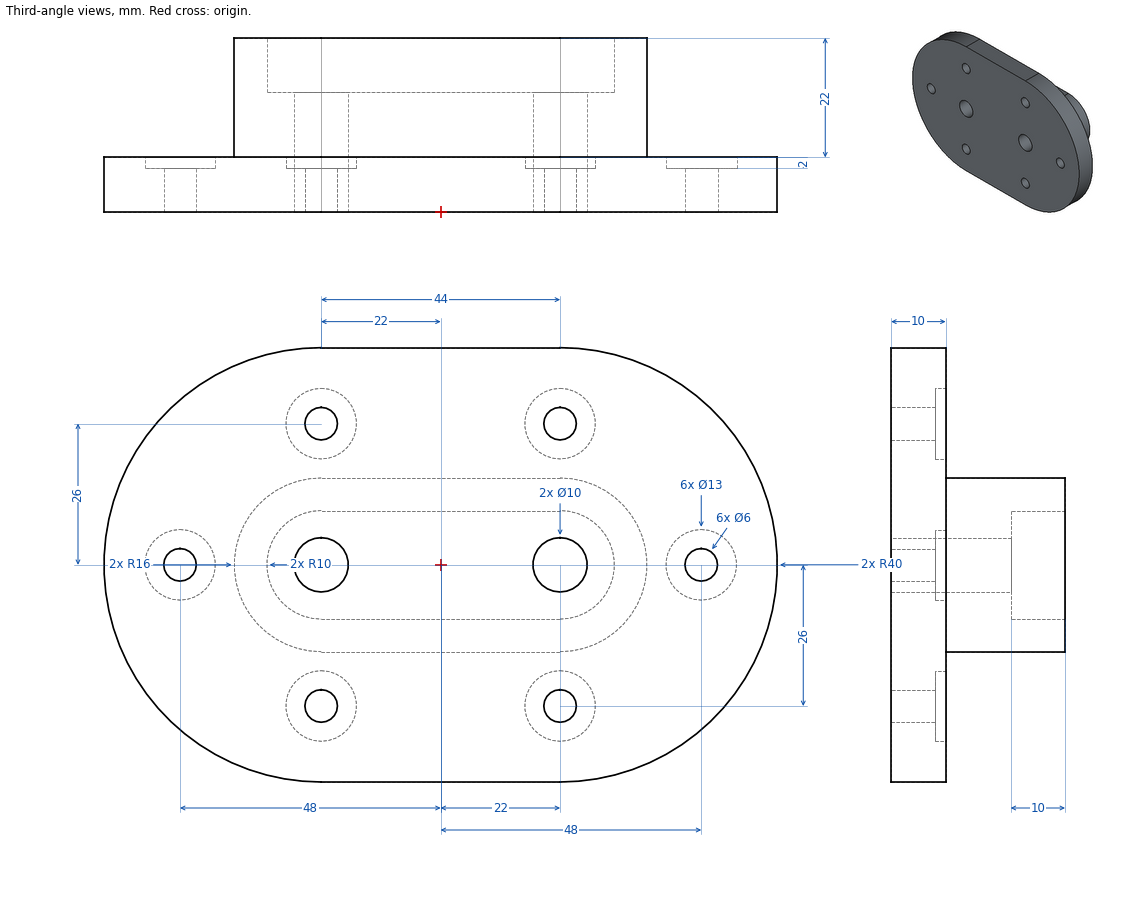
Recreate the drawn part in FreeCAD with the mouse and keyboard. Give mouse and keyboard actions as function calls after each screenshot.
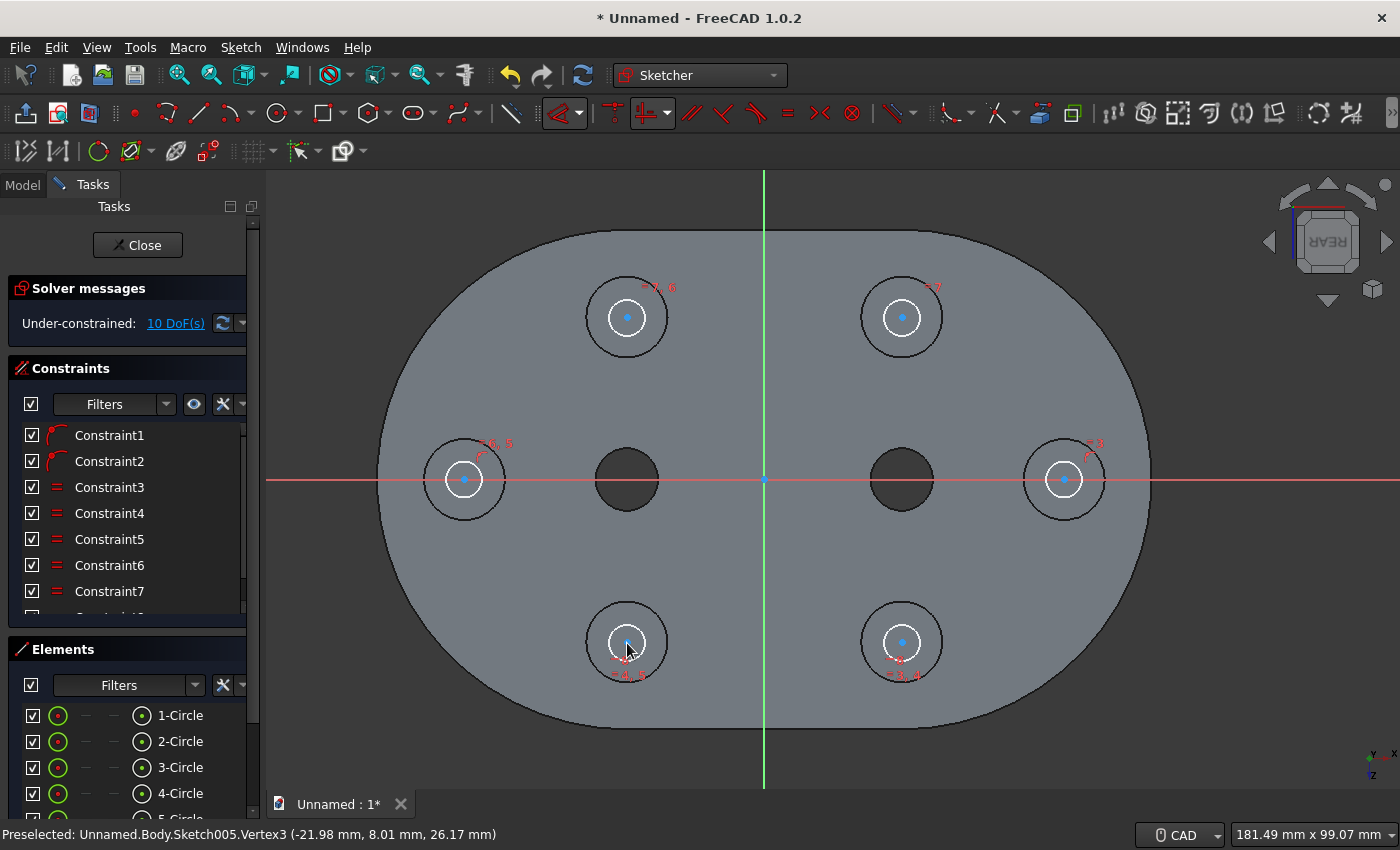
click(627, 643)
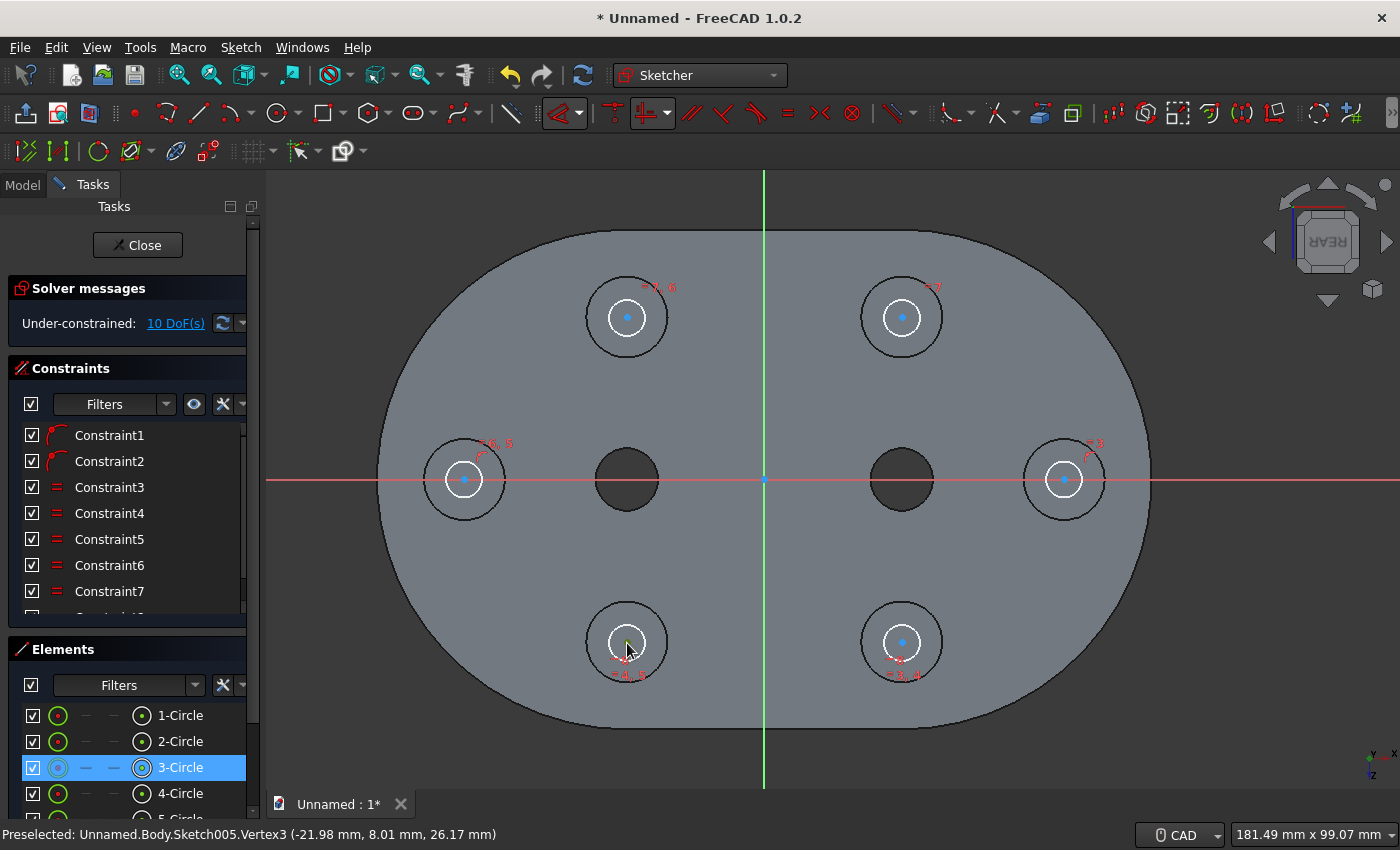
click(627, 318)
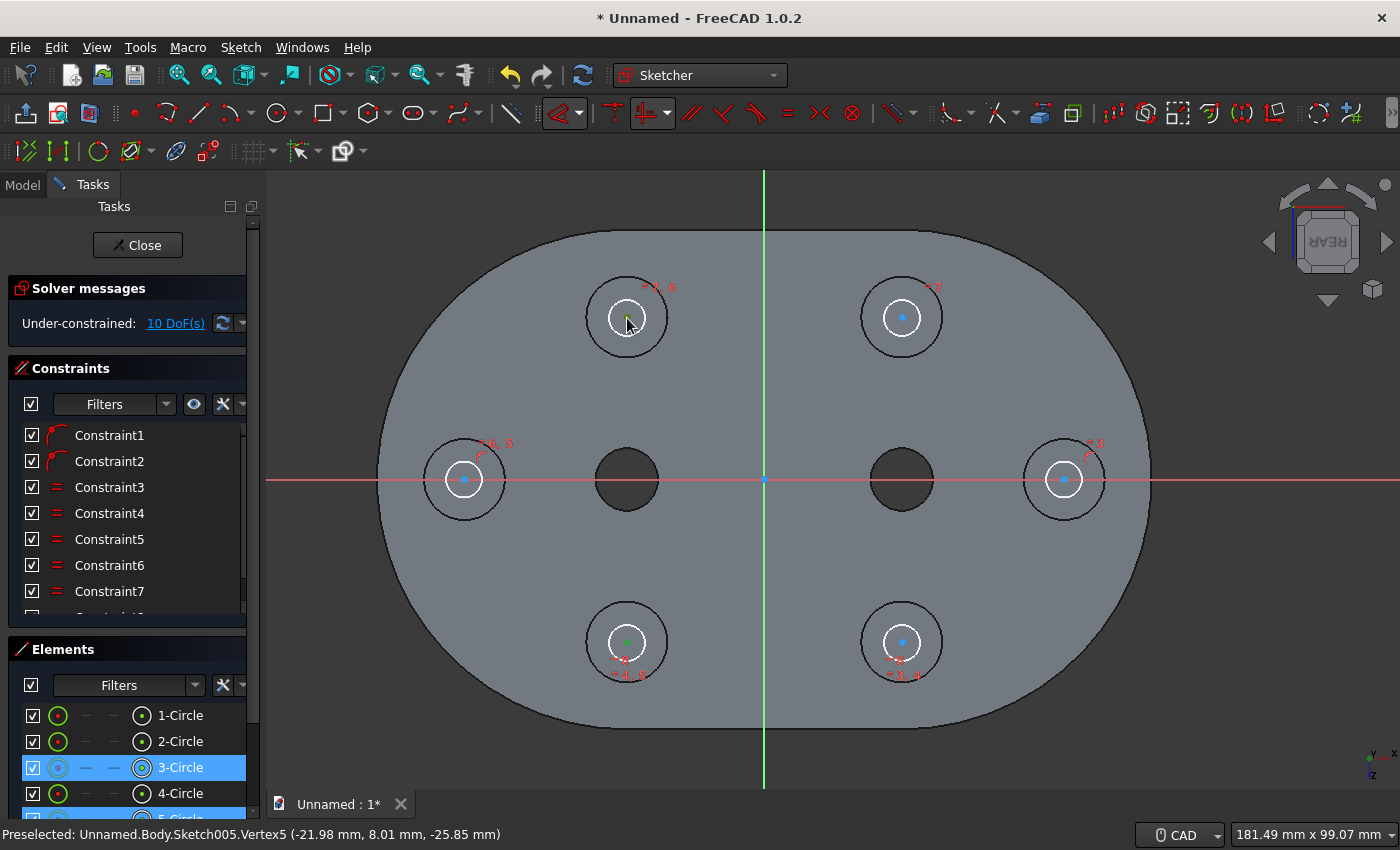
click(670, 114)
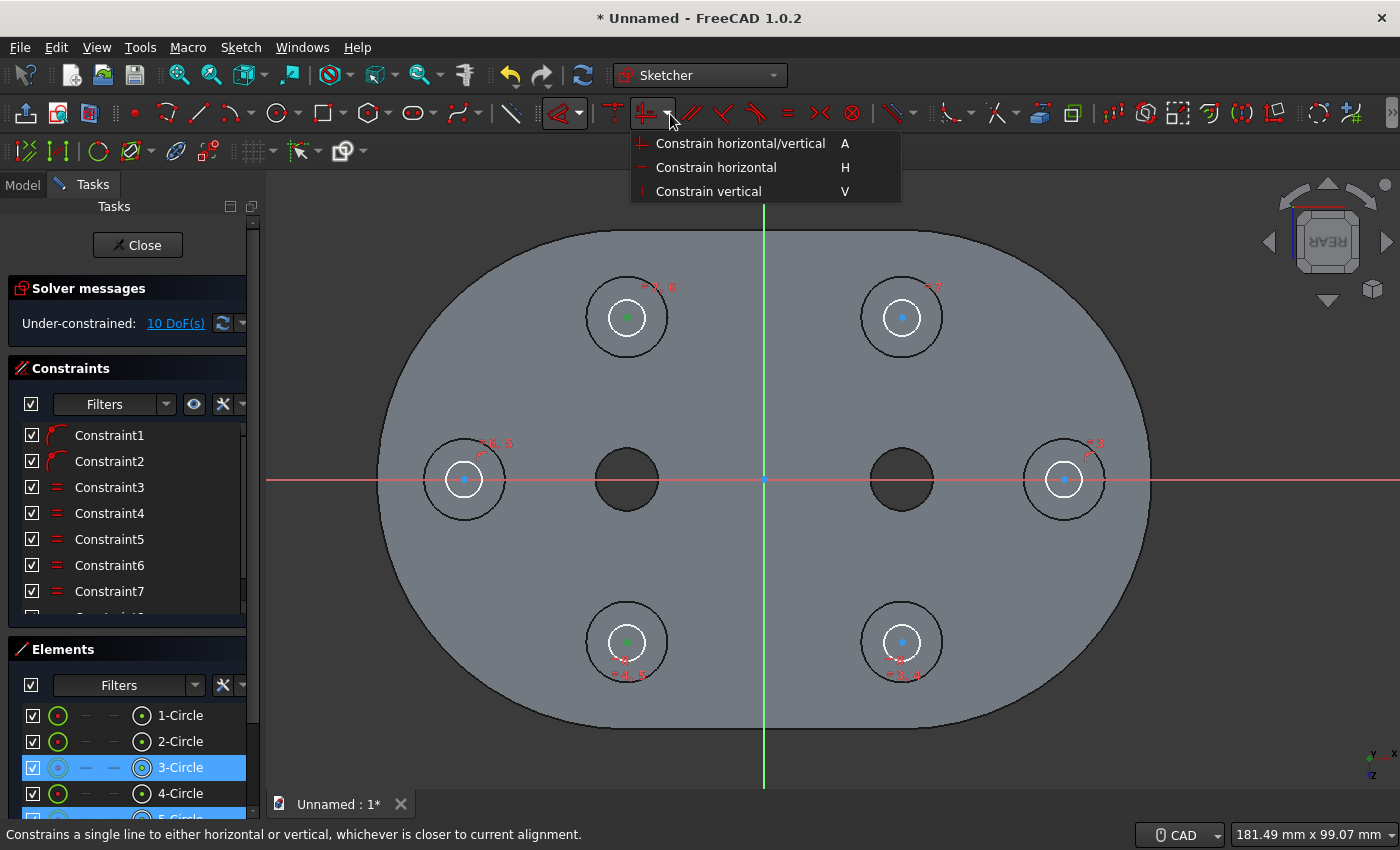
click(766, 191)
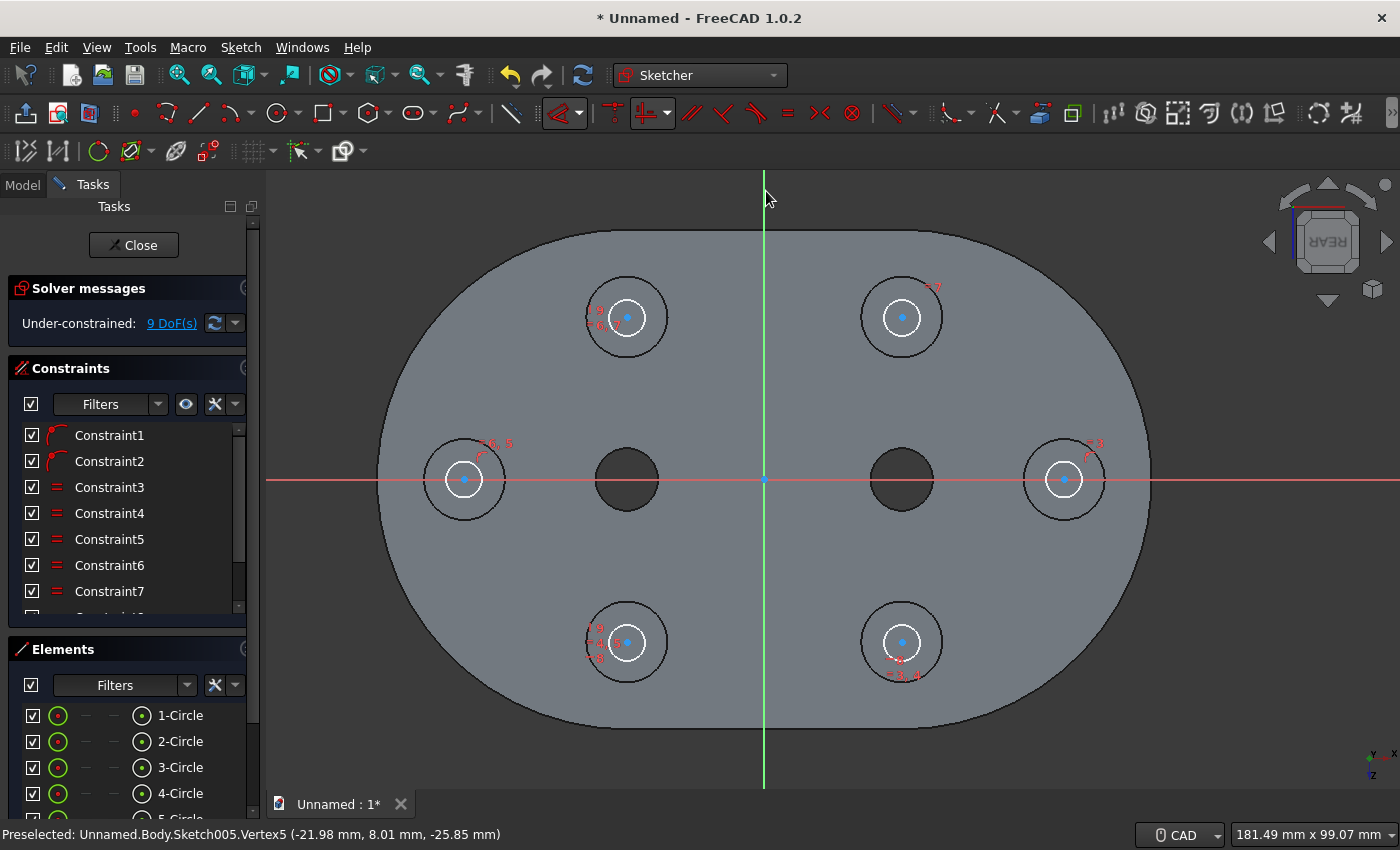
click(902, 643)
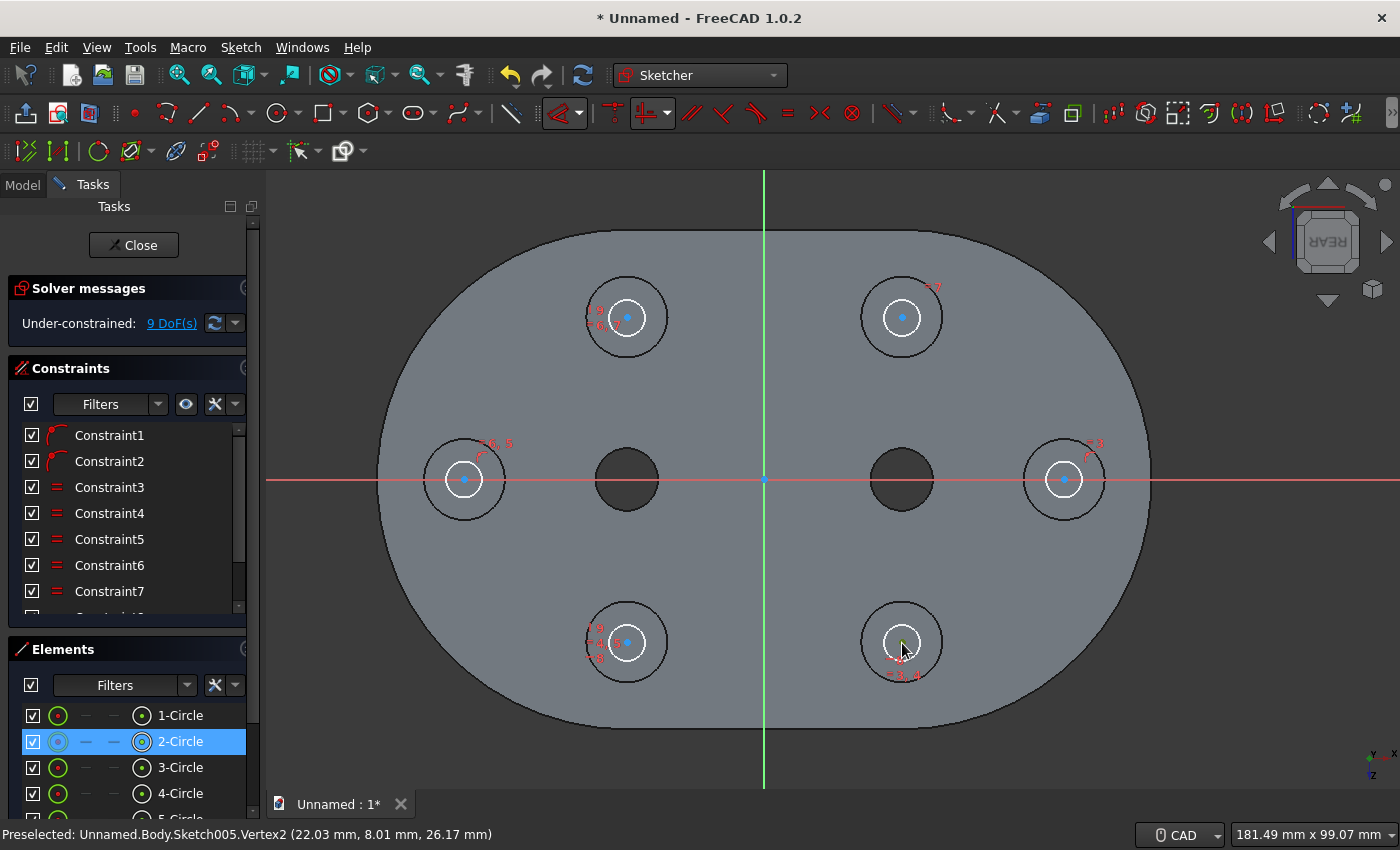
click(902, 318)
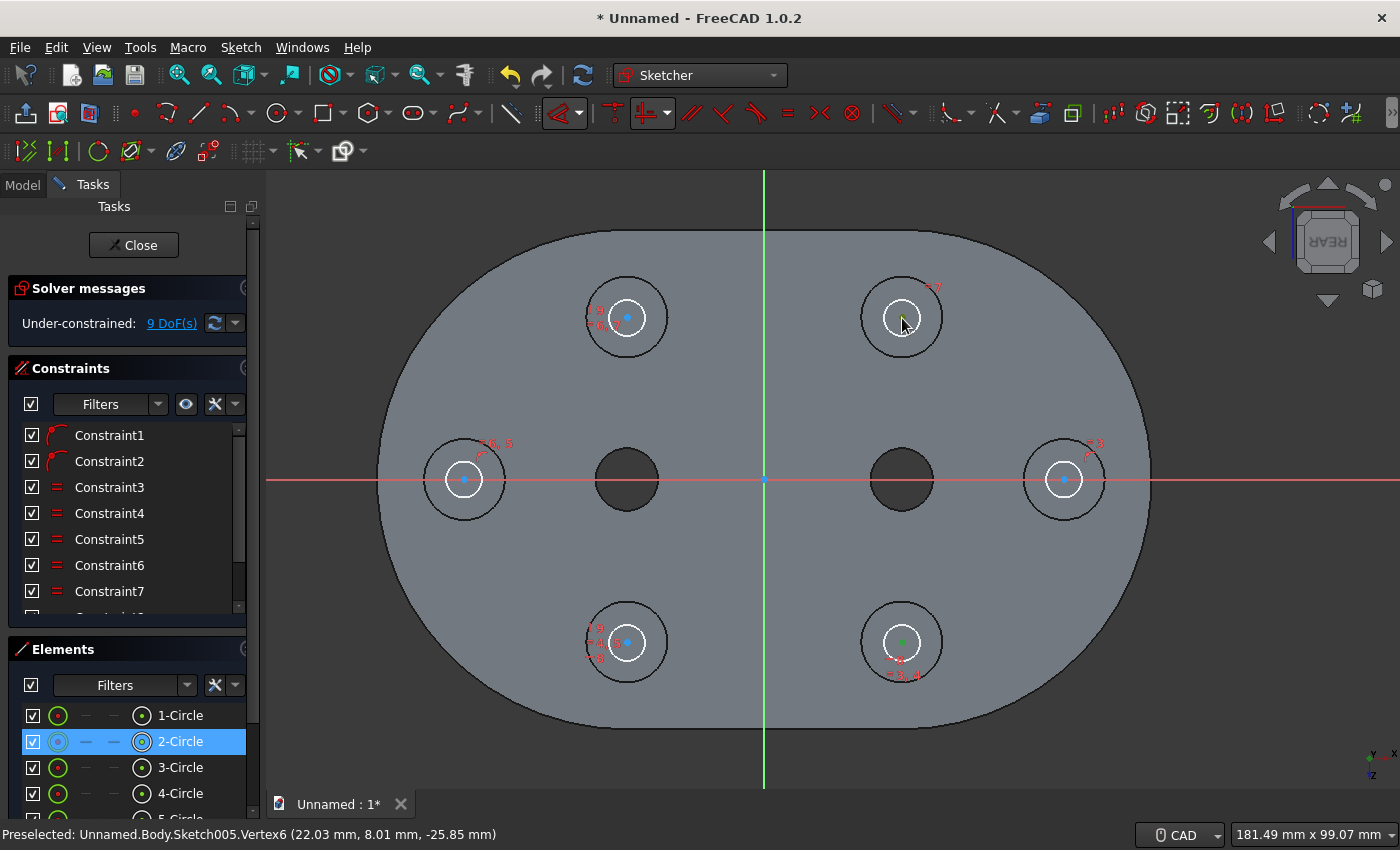
key(v)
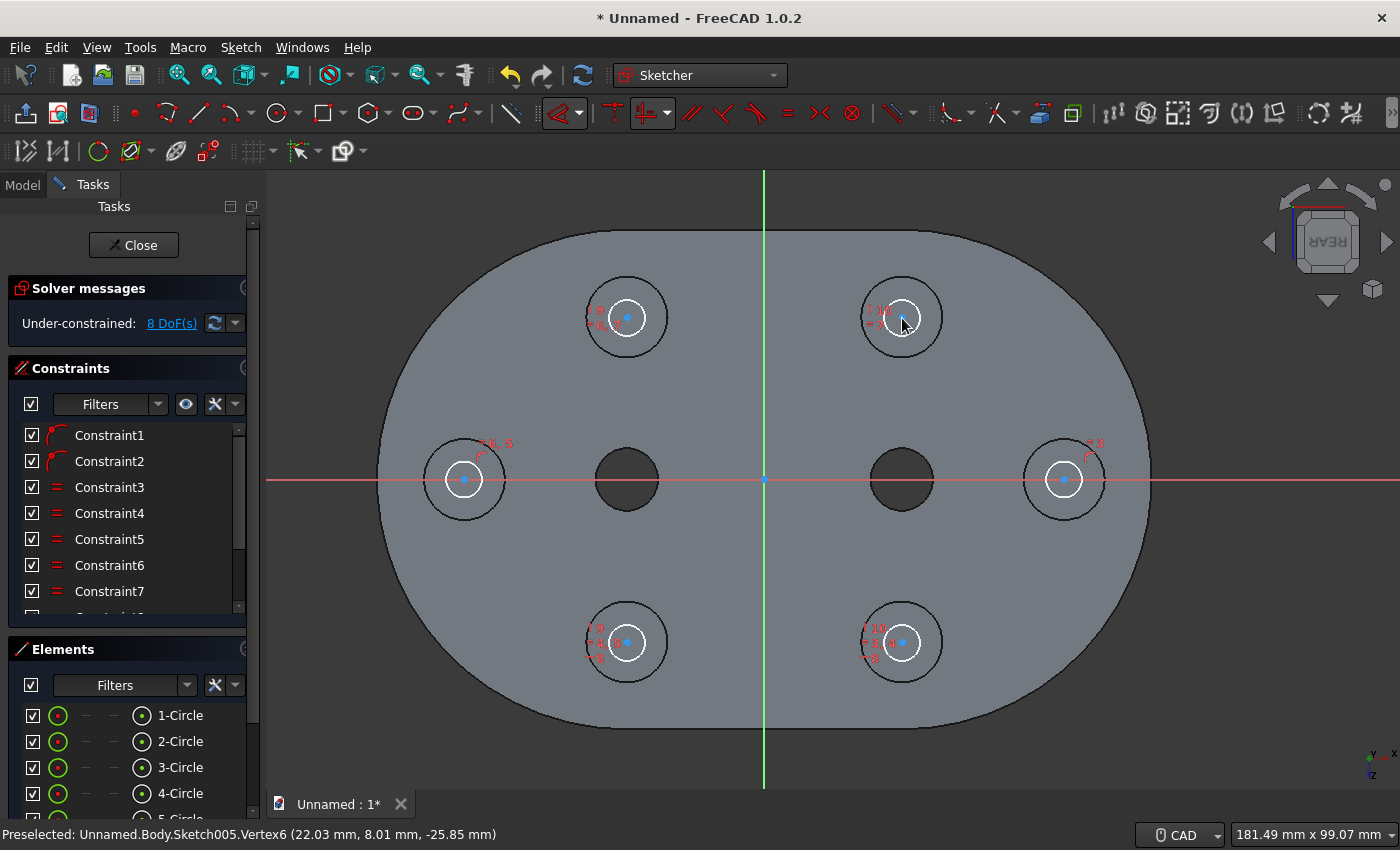
click(627, 318)